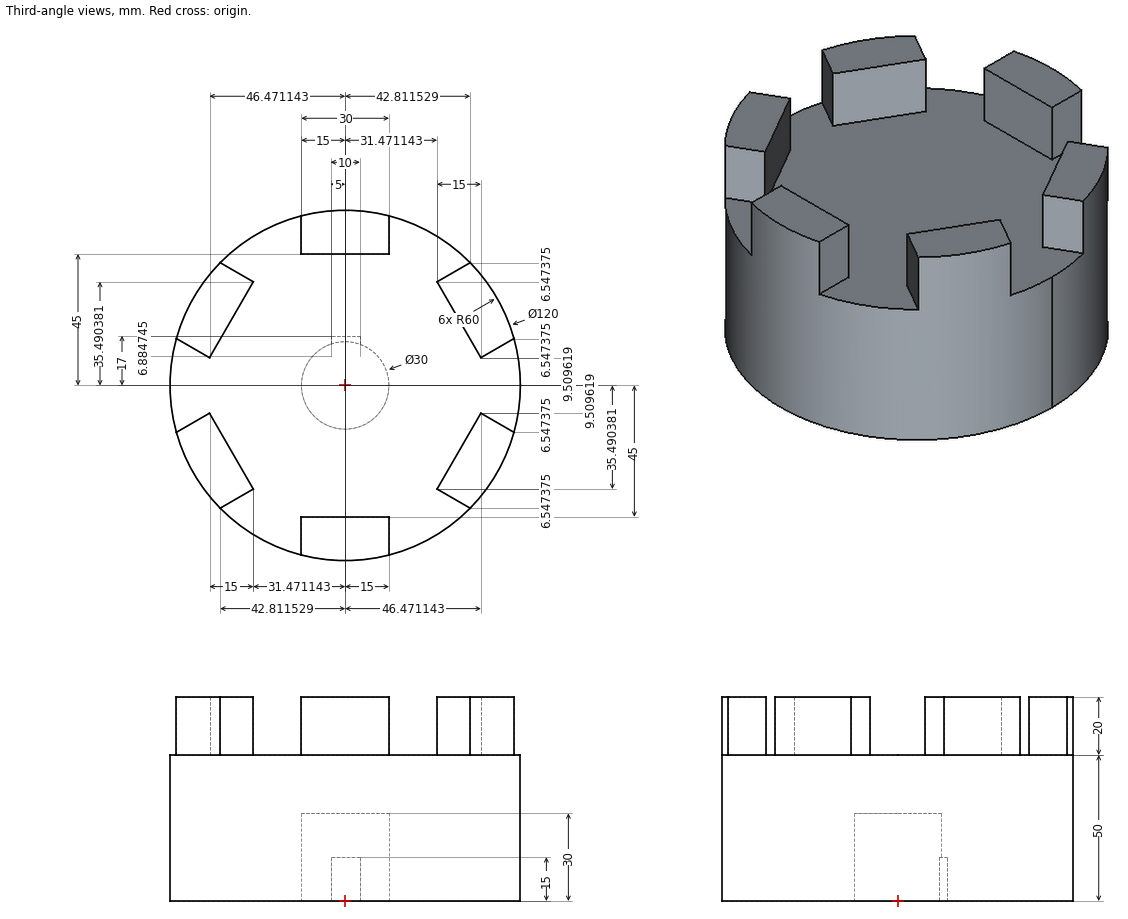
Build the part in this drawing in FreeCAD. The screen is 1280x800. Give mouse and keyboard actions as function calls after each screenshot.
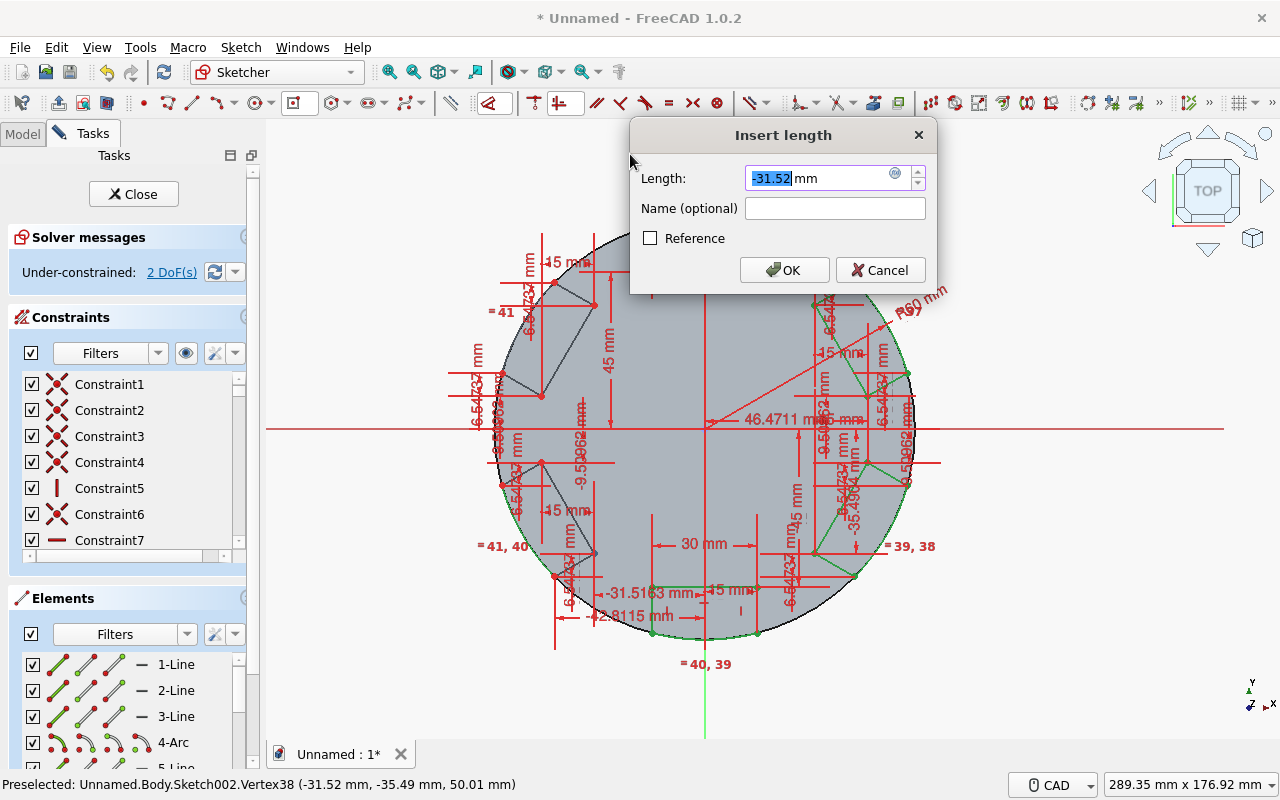
text(-31.471143)
key(Return)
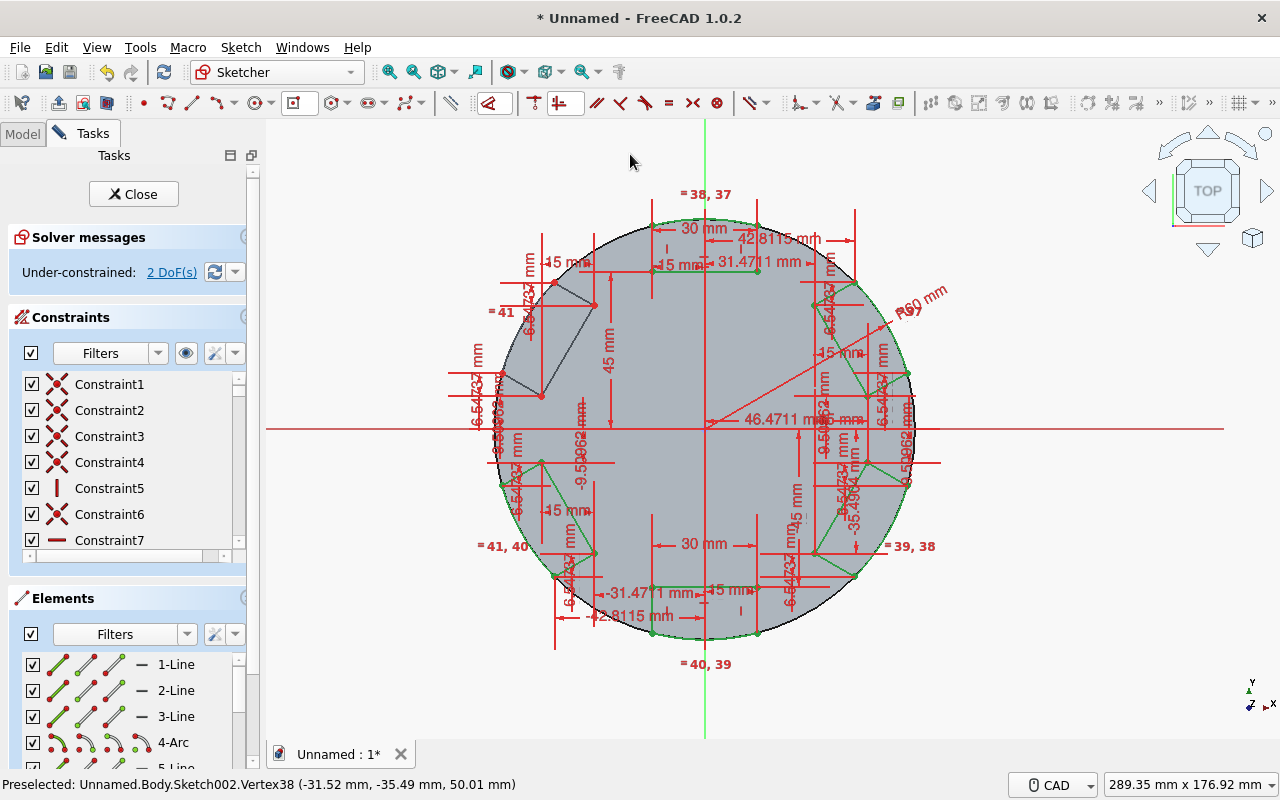
click(542, 396)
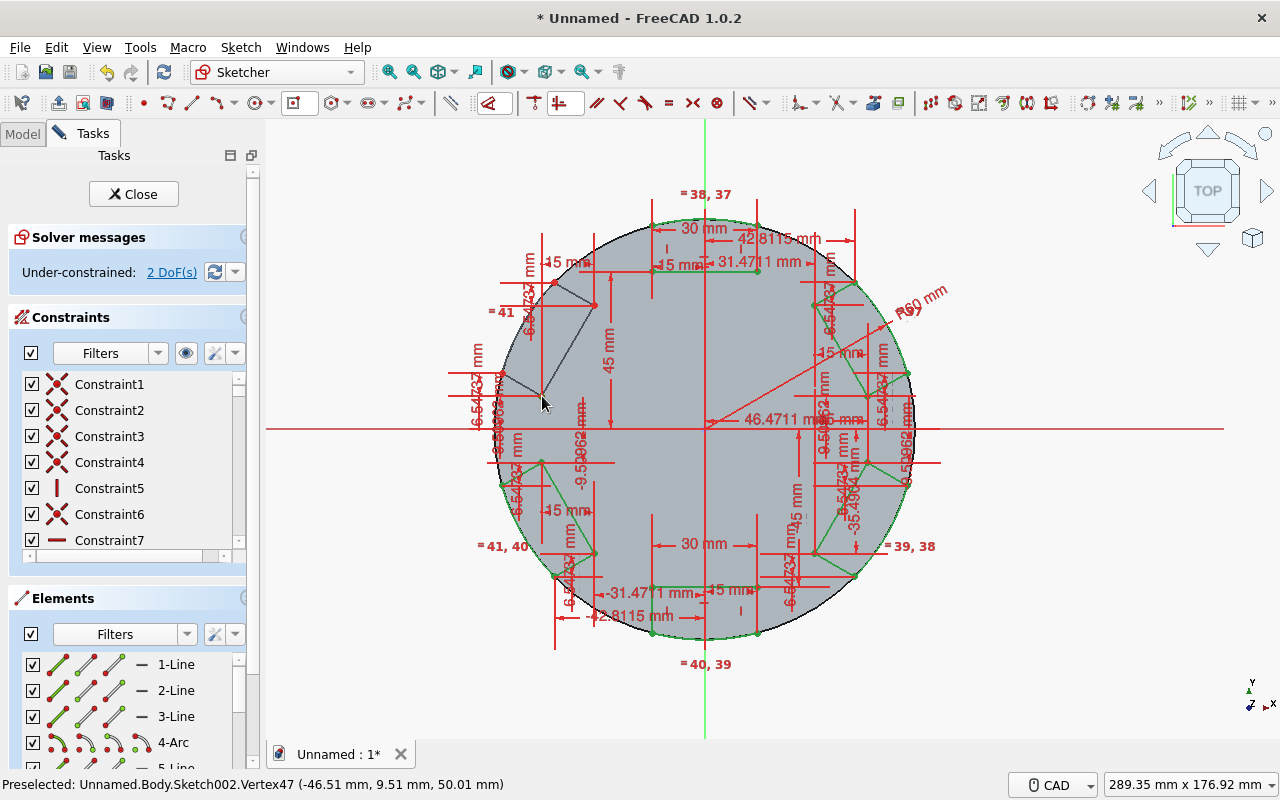
key(l)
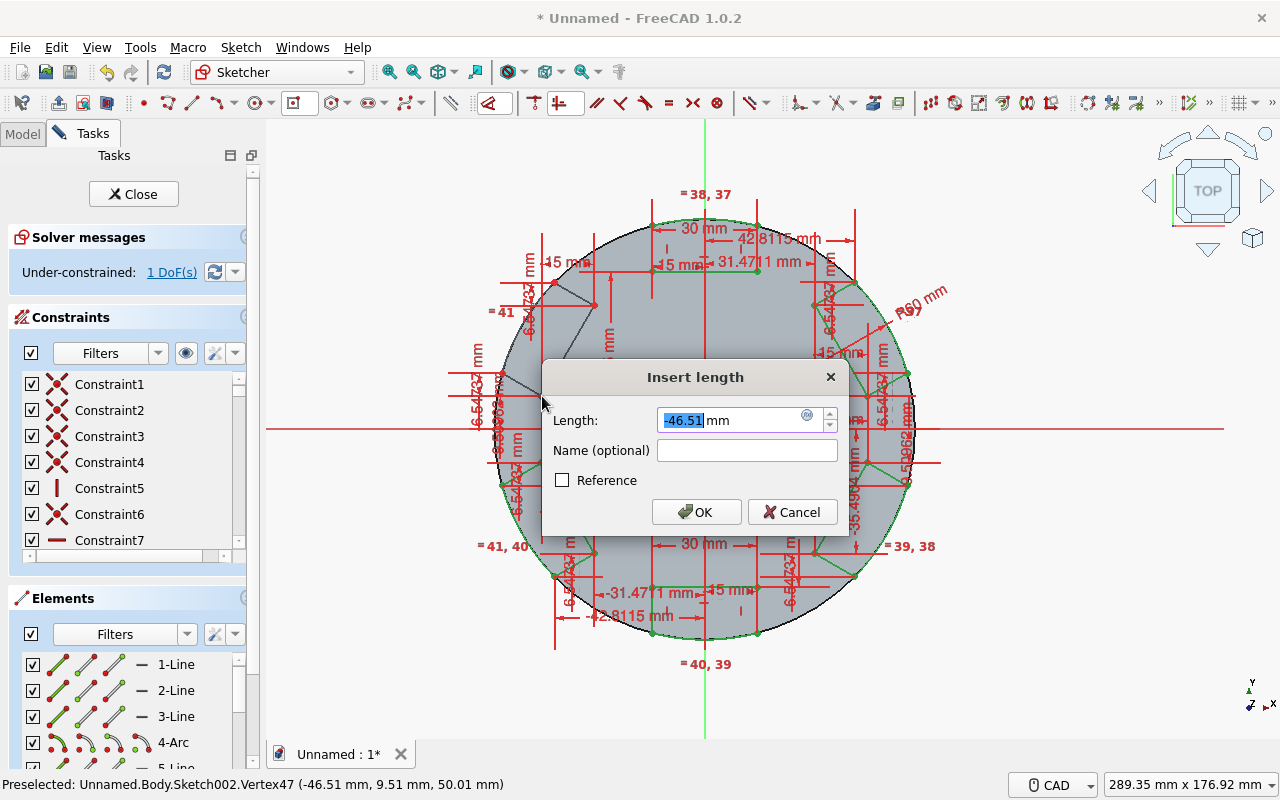
text(-46.471143)
key(Return)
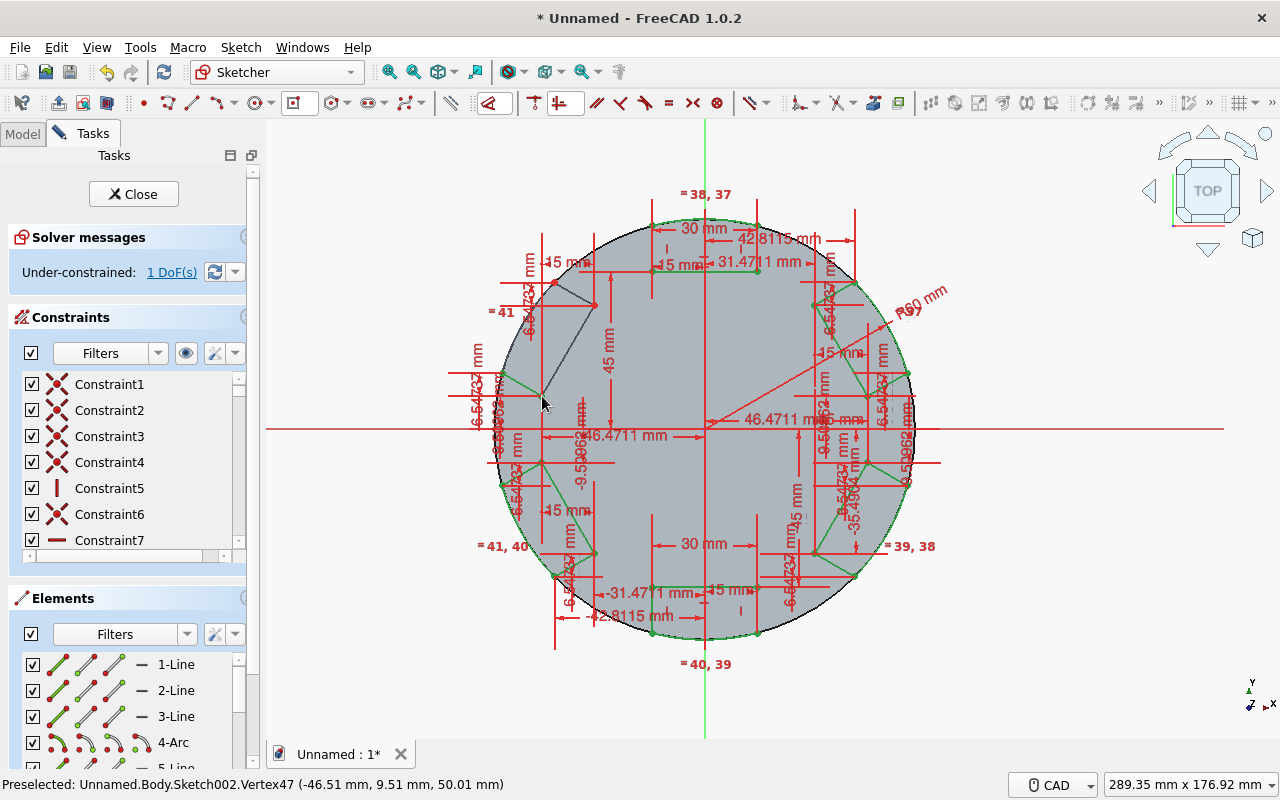
click(594, 306)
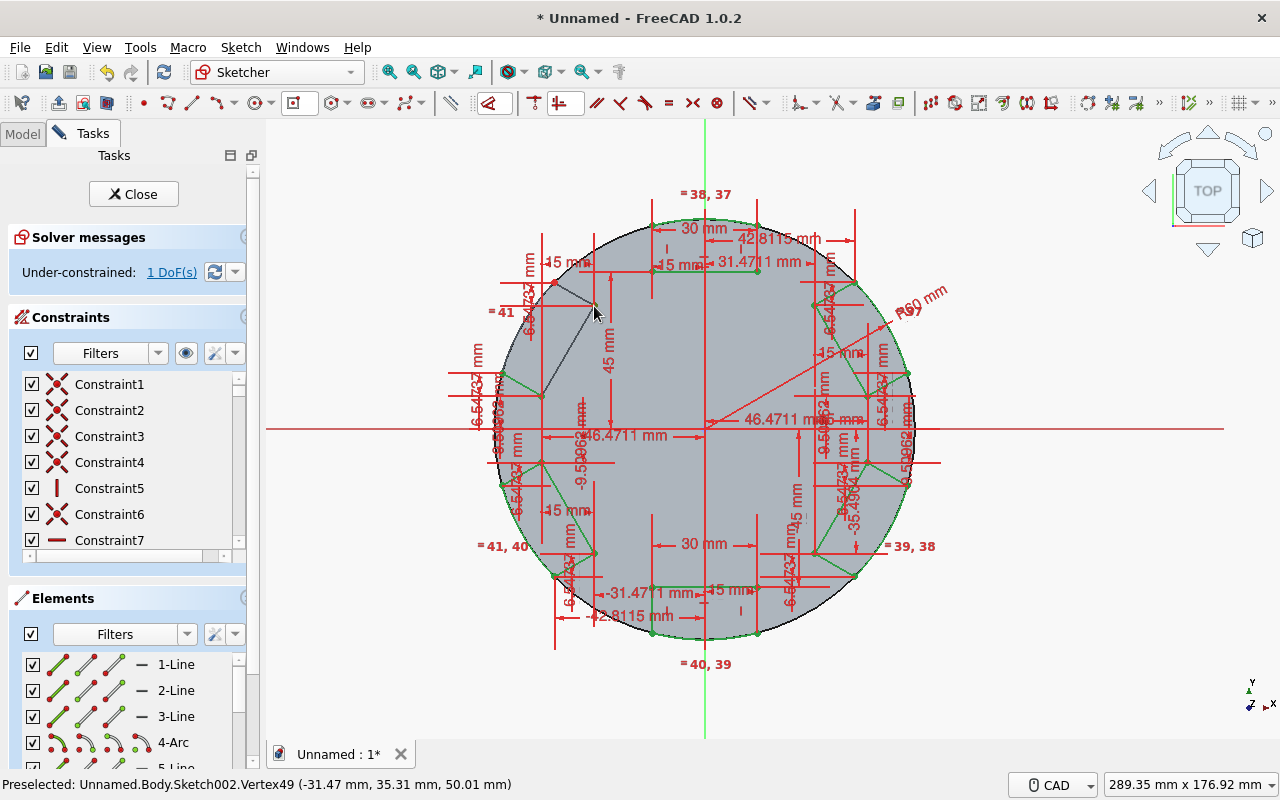
key(i)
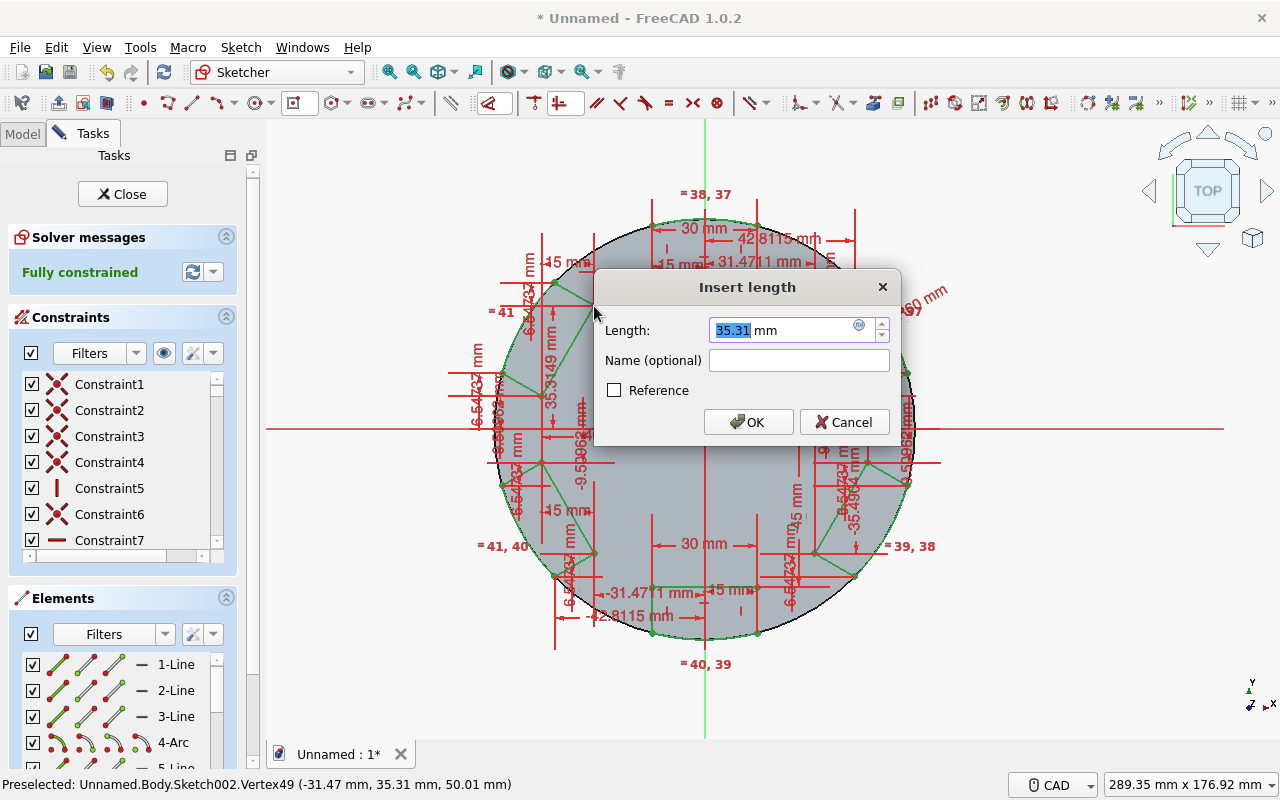
text(35.490381)
key(Return)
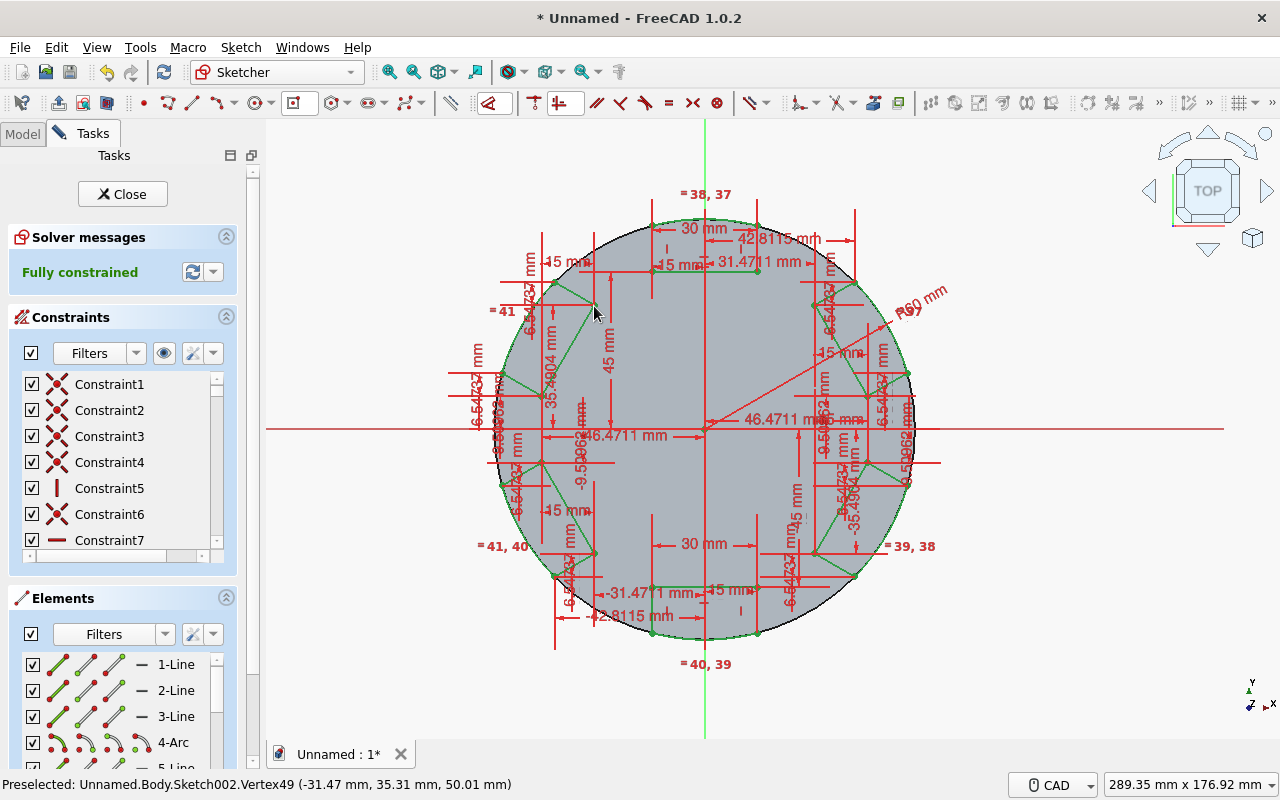
click(123, 194)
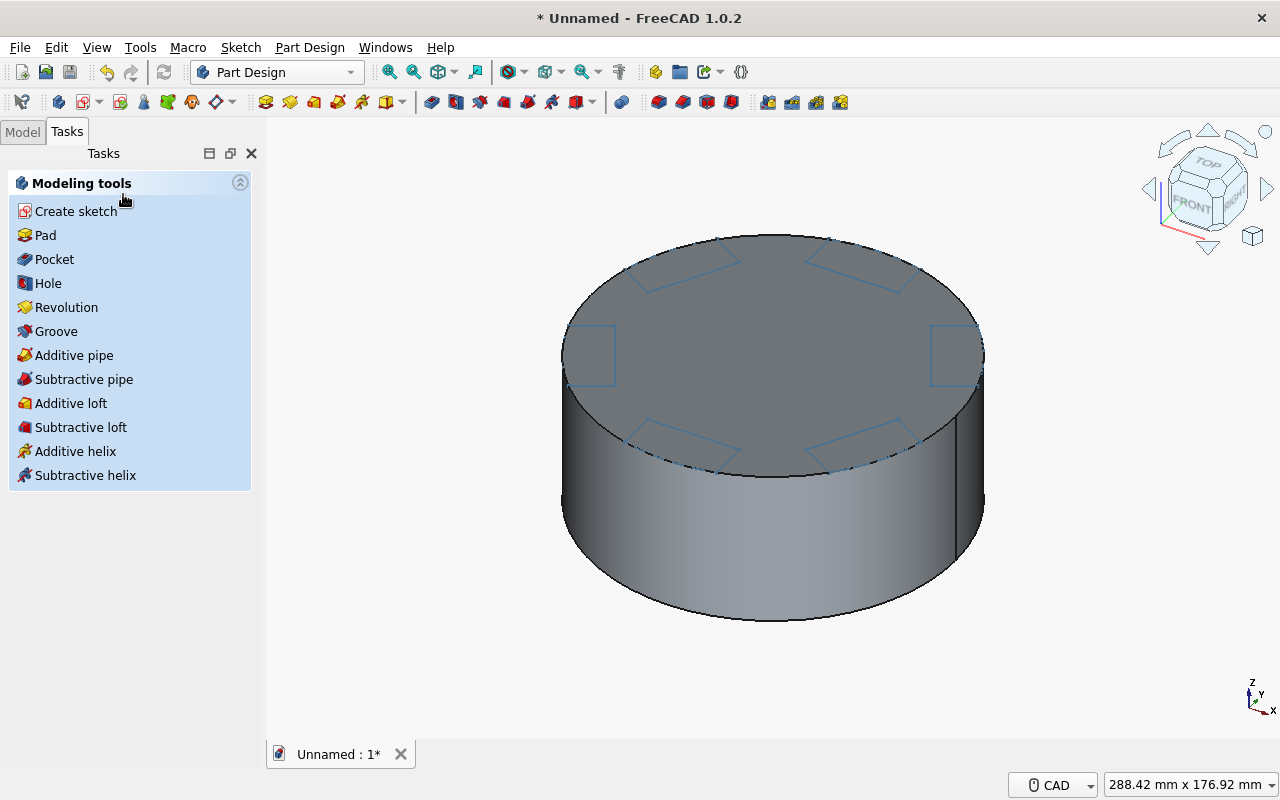
click(266, 102)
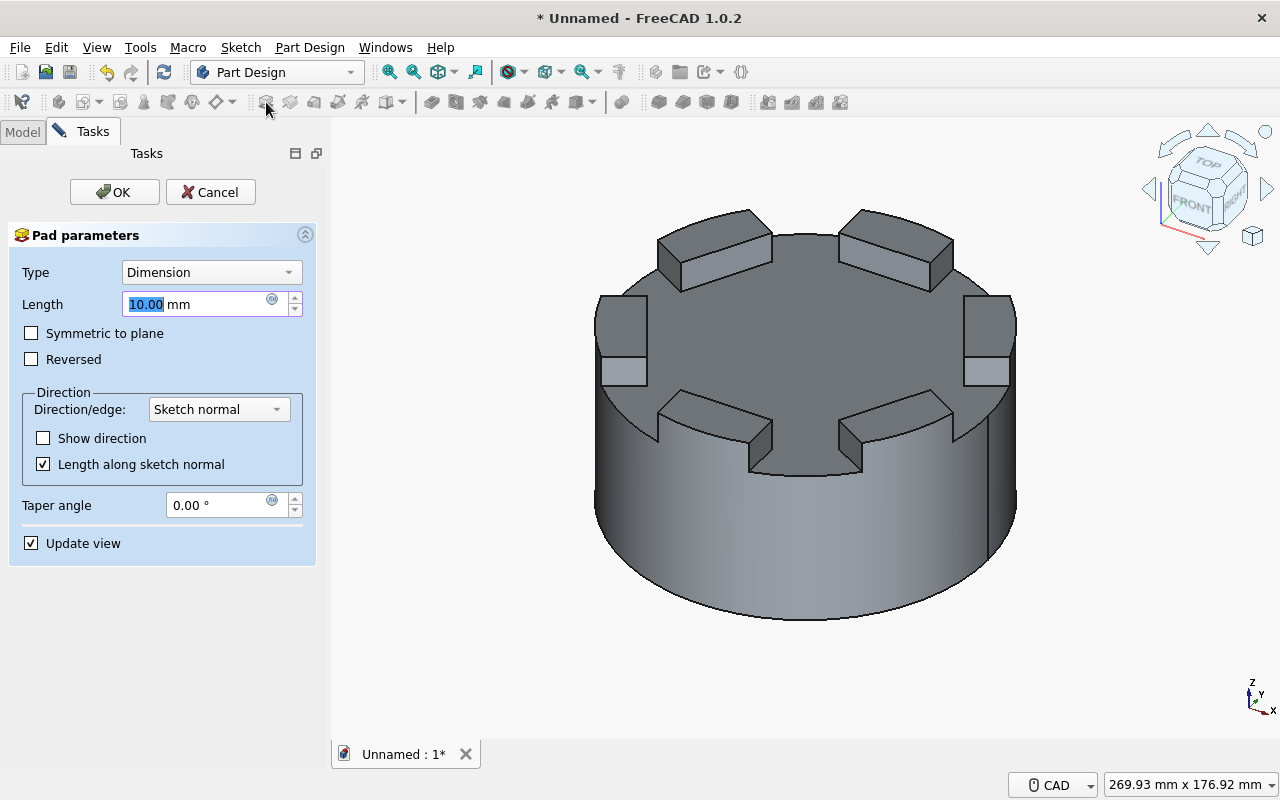
text(20)
key(Tab)